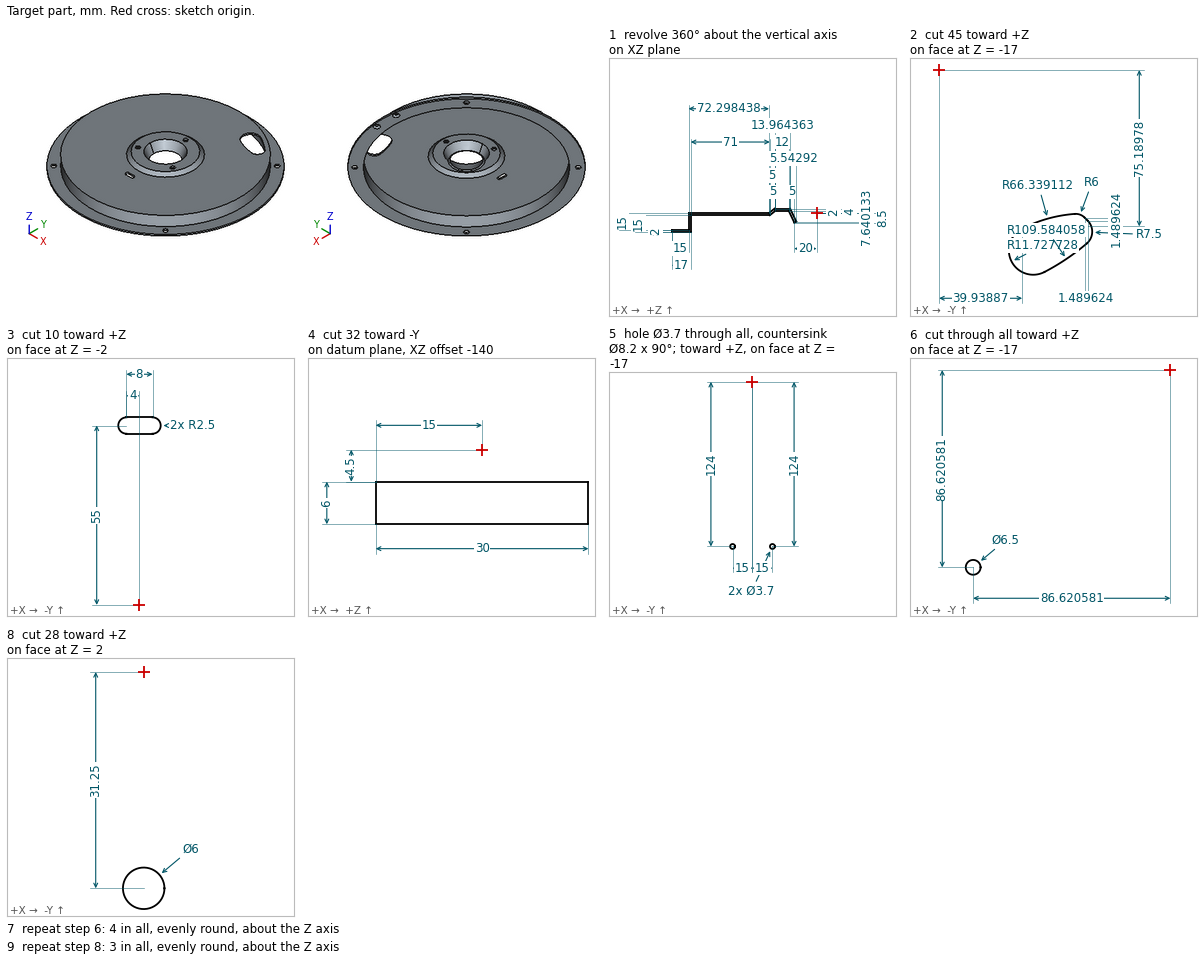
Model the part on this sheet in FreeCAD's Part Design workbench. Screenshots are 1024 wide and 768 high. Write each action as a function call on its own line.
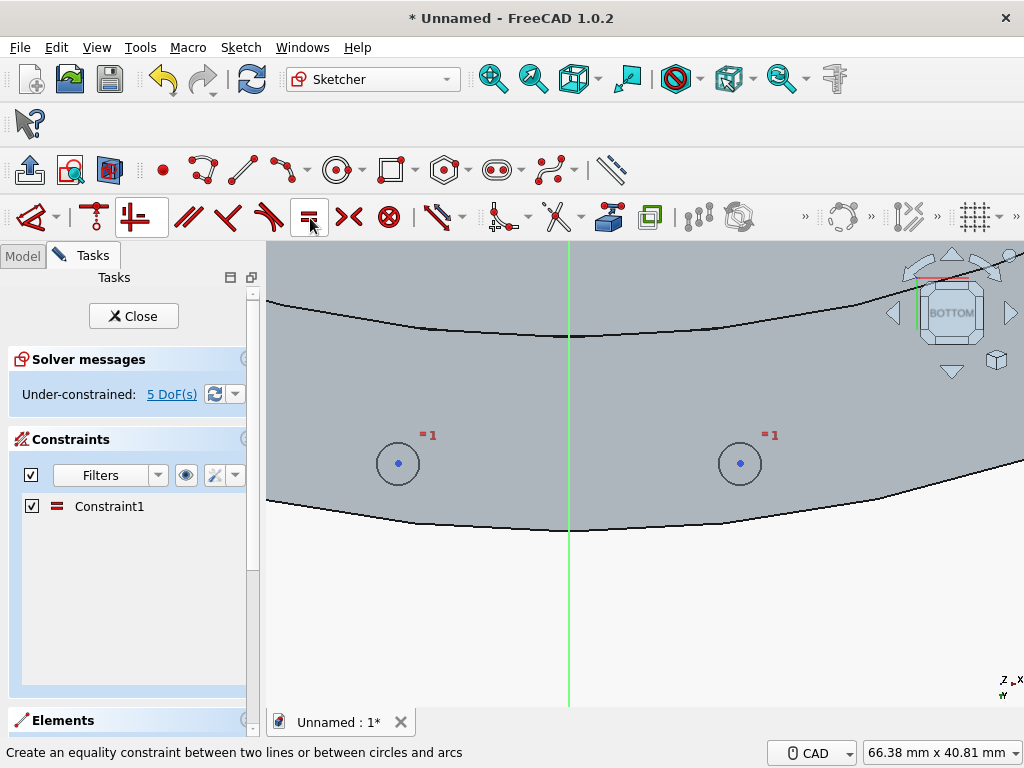
click(32, 218)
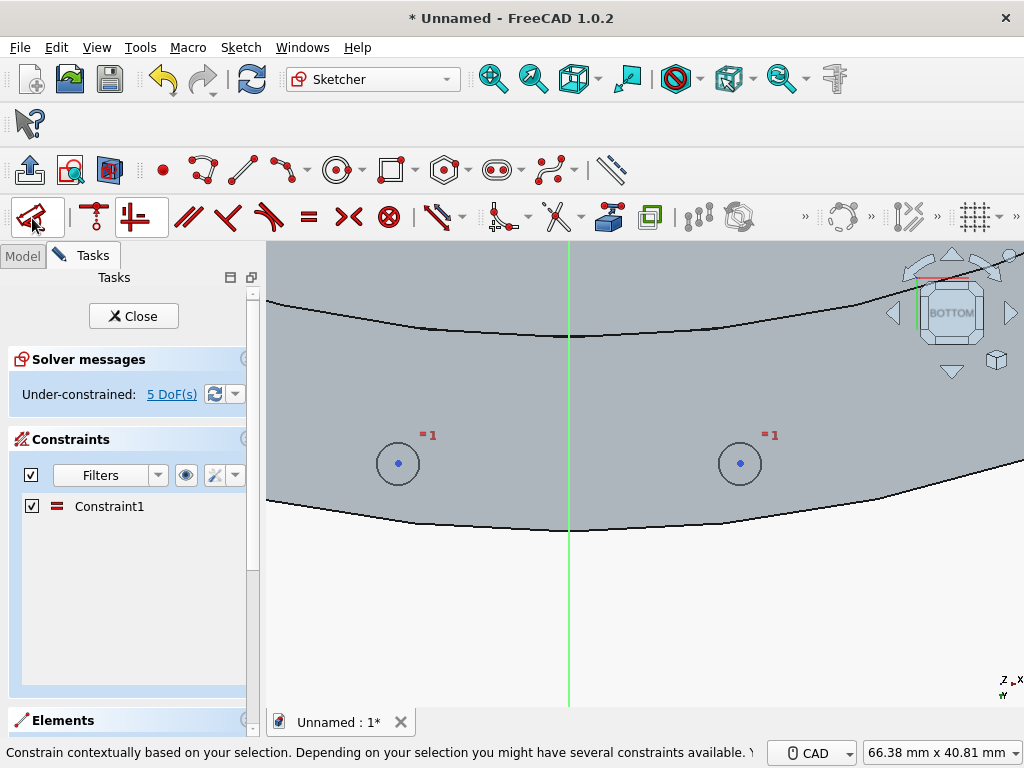
click(755, 449)
click(778, 426)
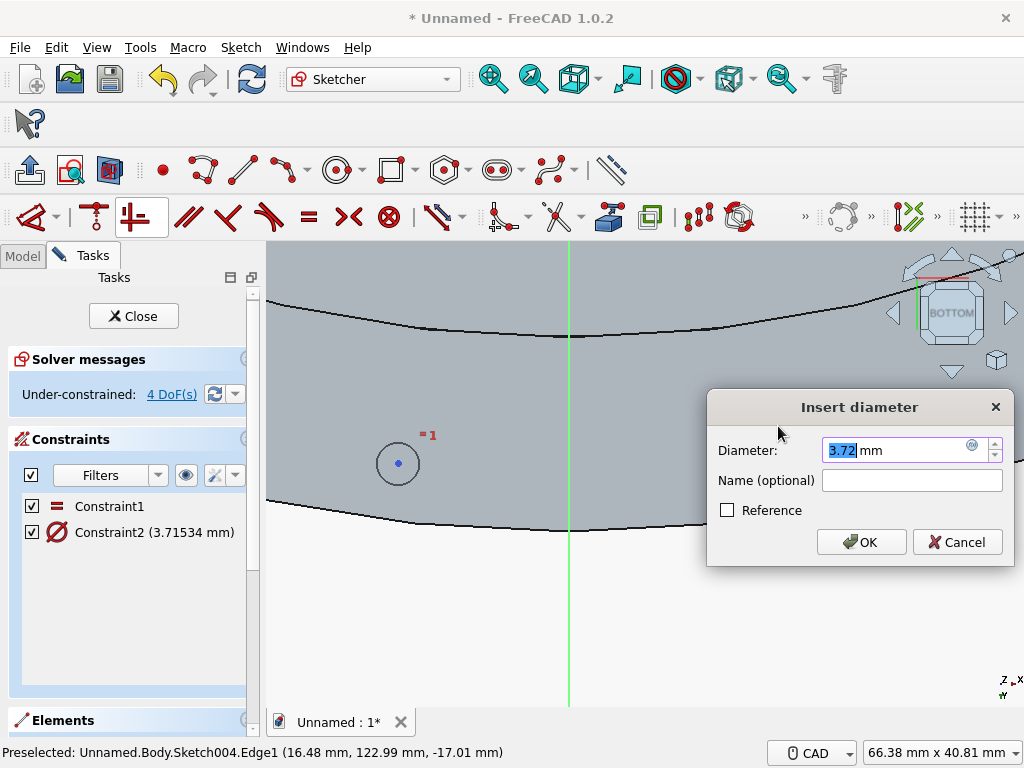
text(3.7)
key(Return)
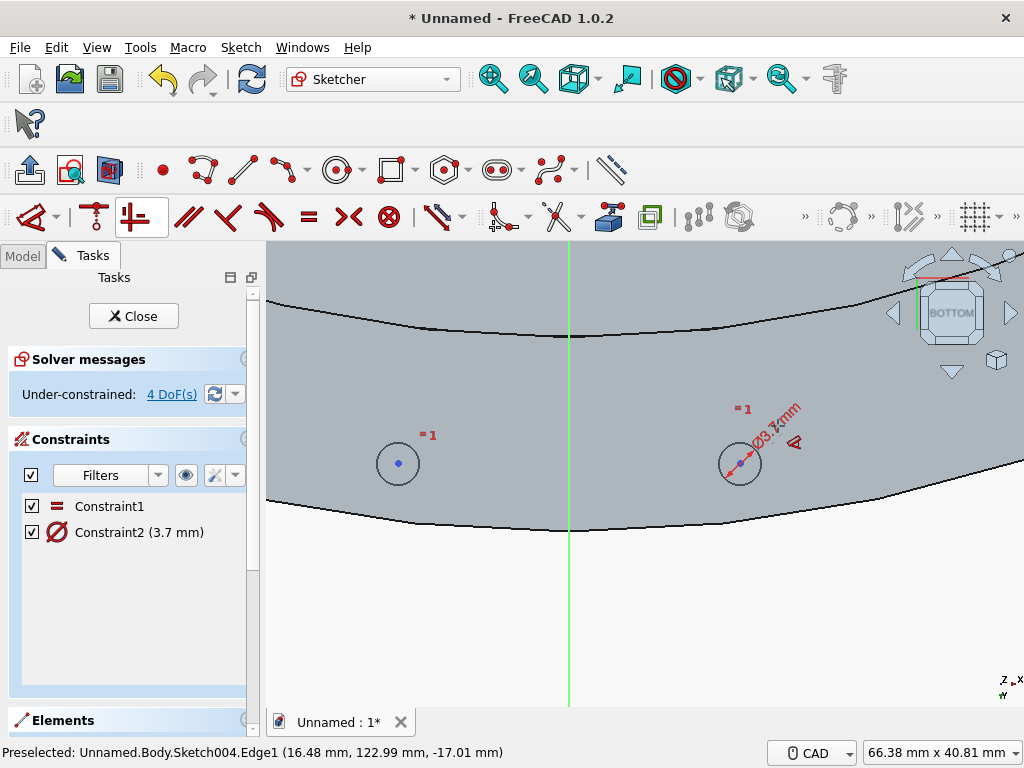
click(740, 464)
click(654, 498)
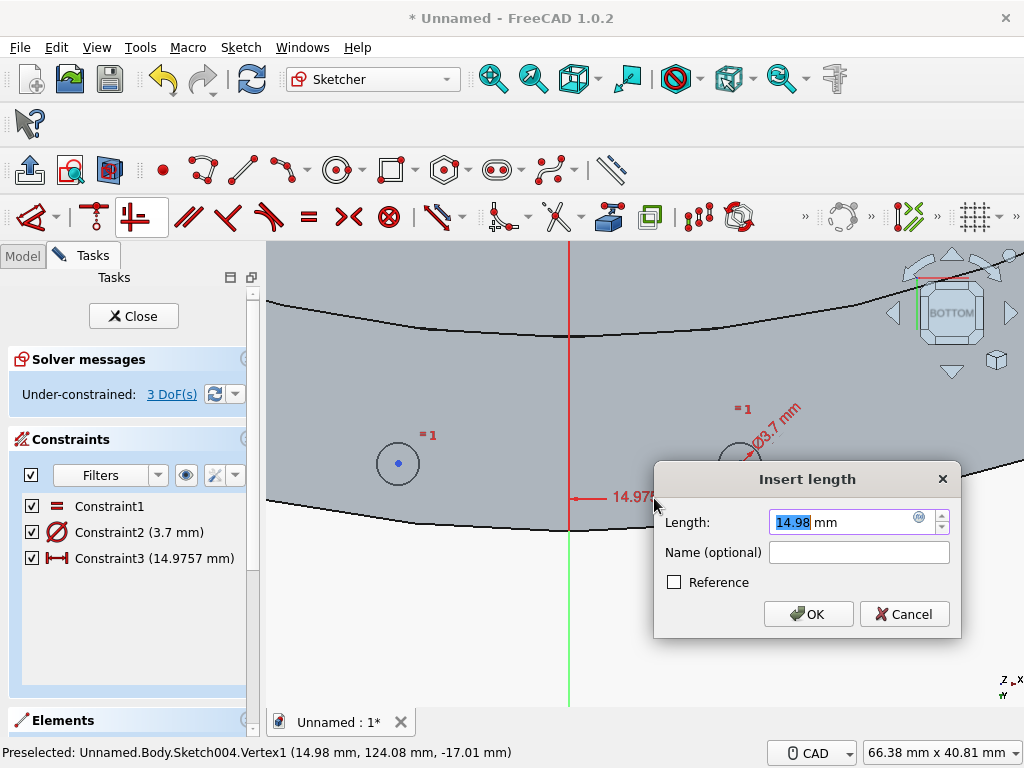
text(15)
key(Return)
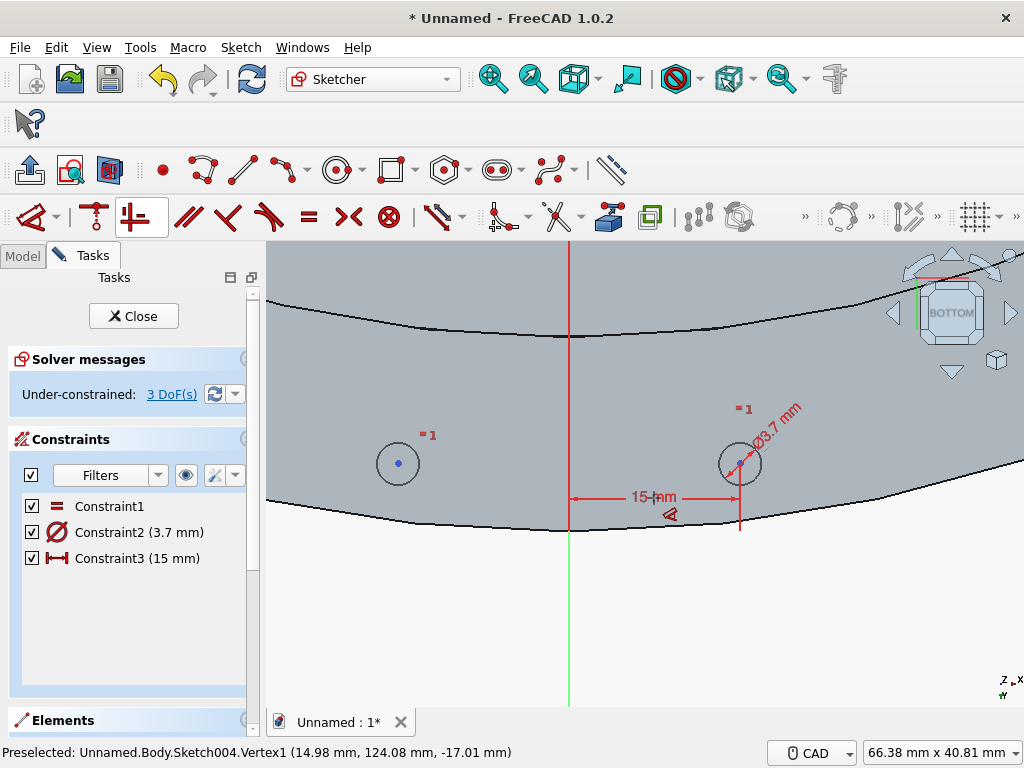
click(398, 464)
click(483, 498)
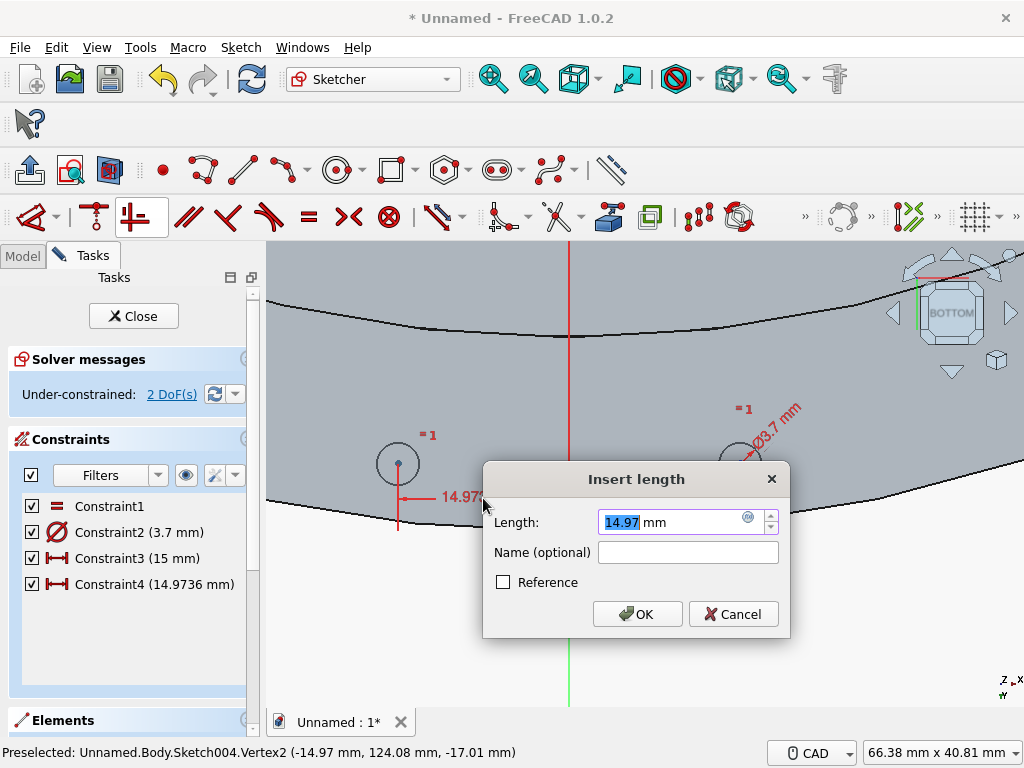
text(15)
key(Return)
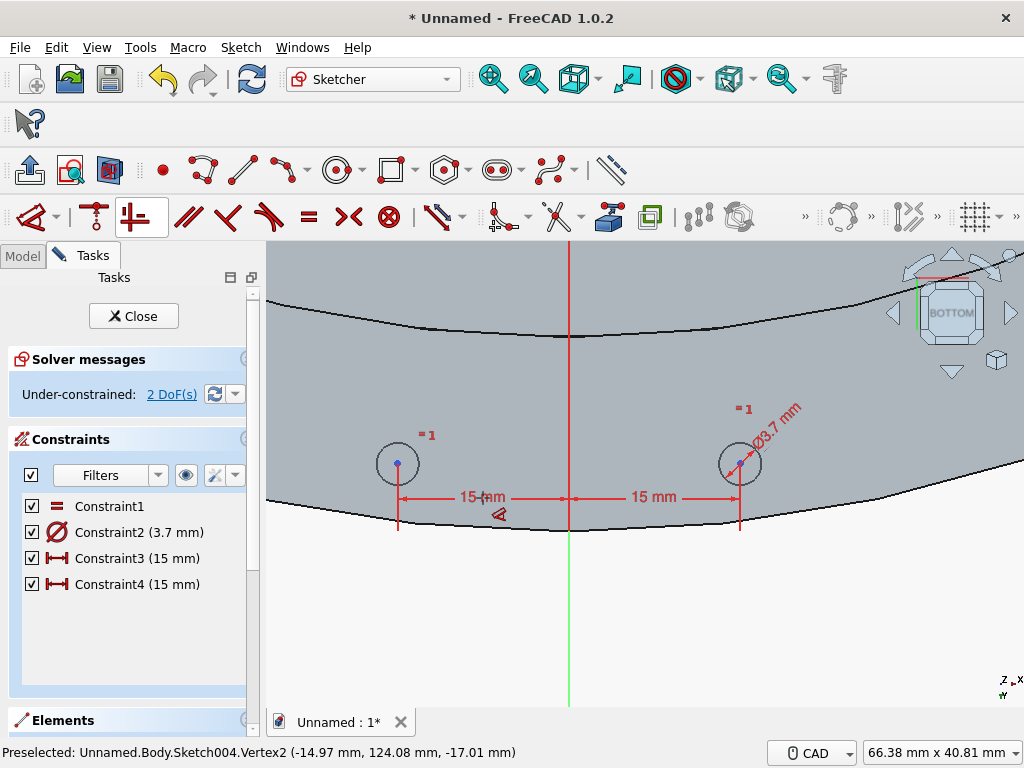
click(740, 464)
click(774, 367)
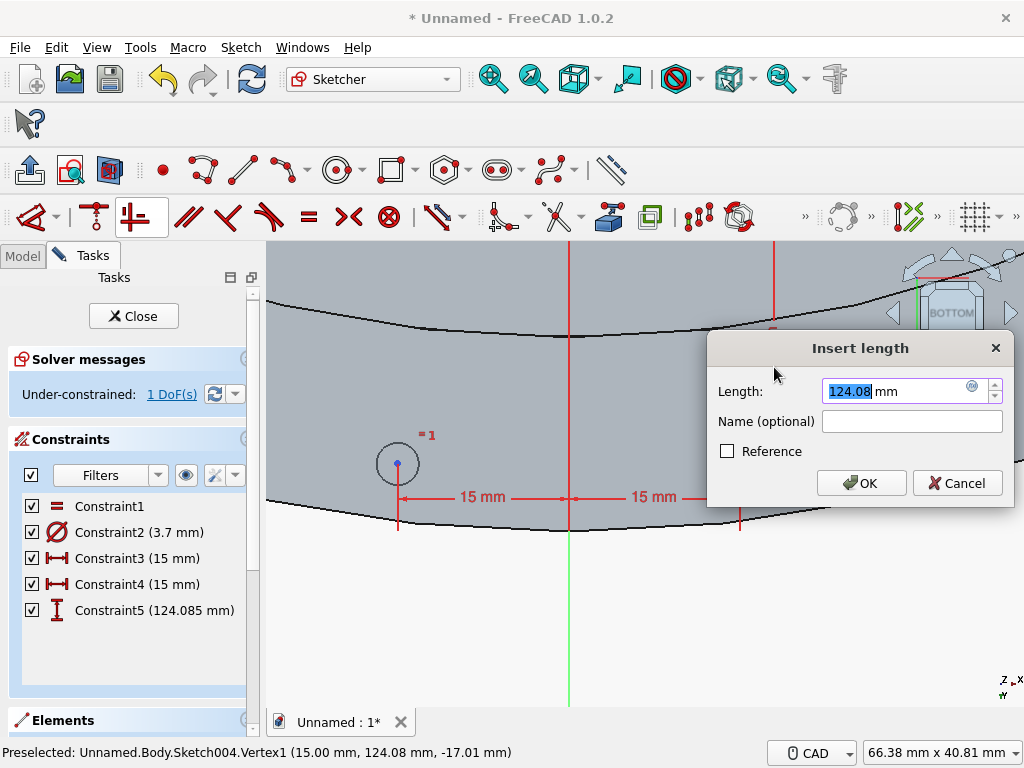
text(124)
key(Return)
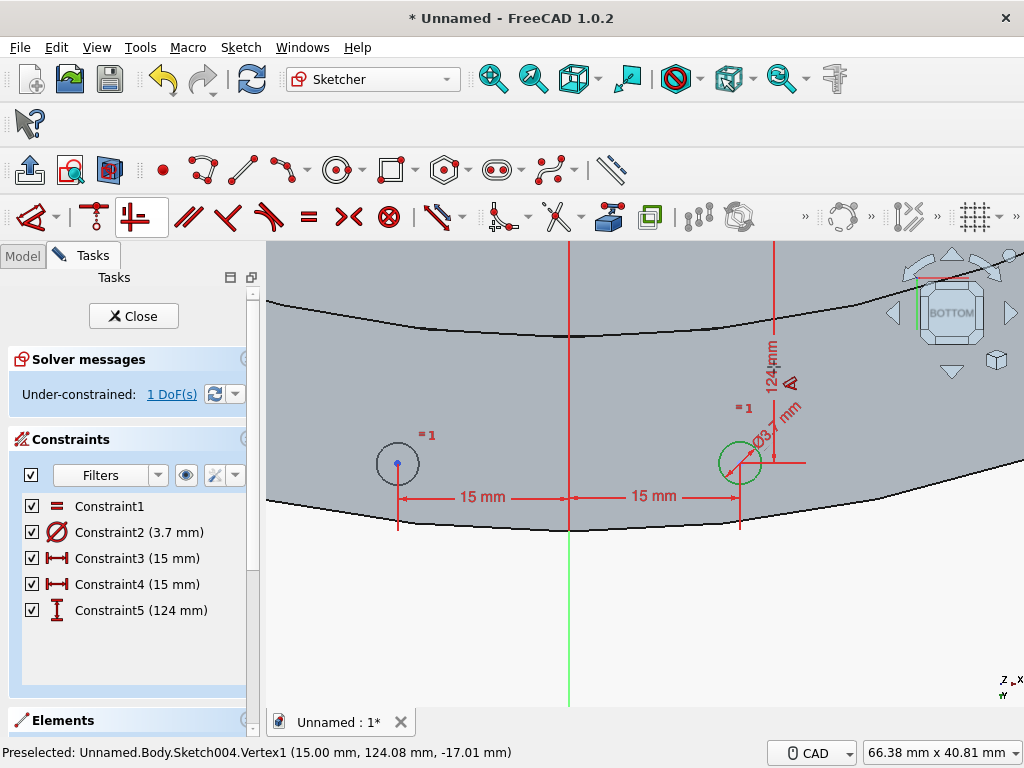
click(398, 464)
click(364, 367)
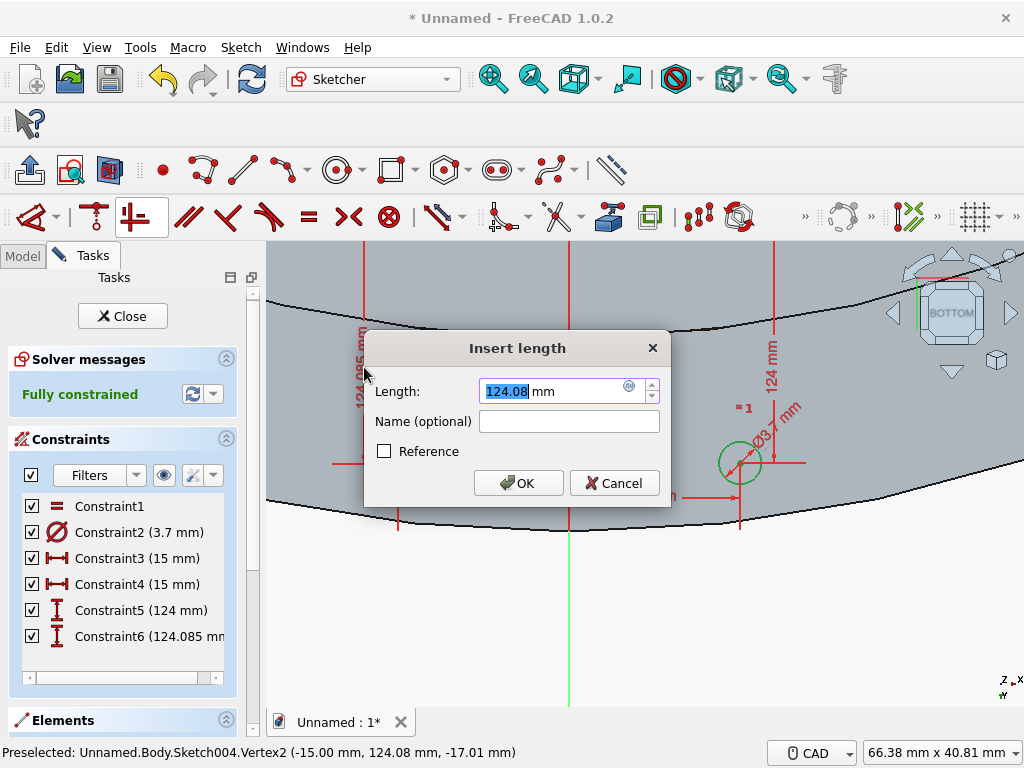
text(124)
key(Return)
key(Escape)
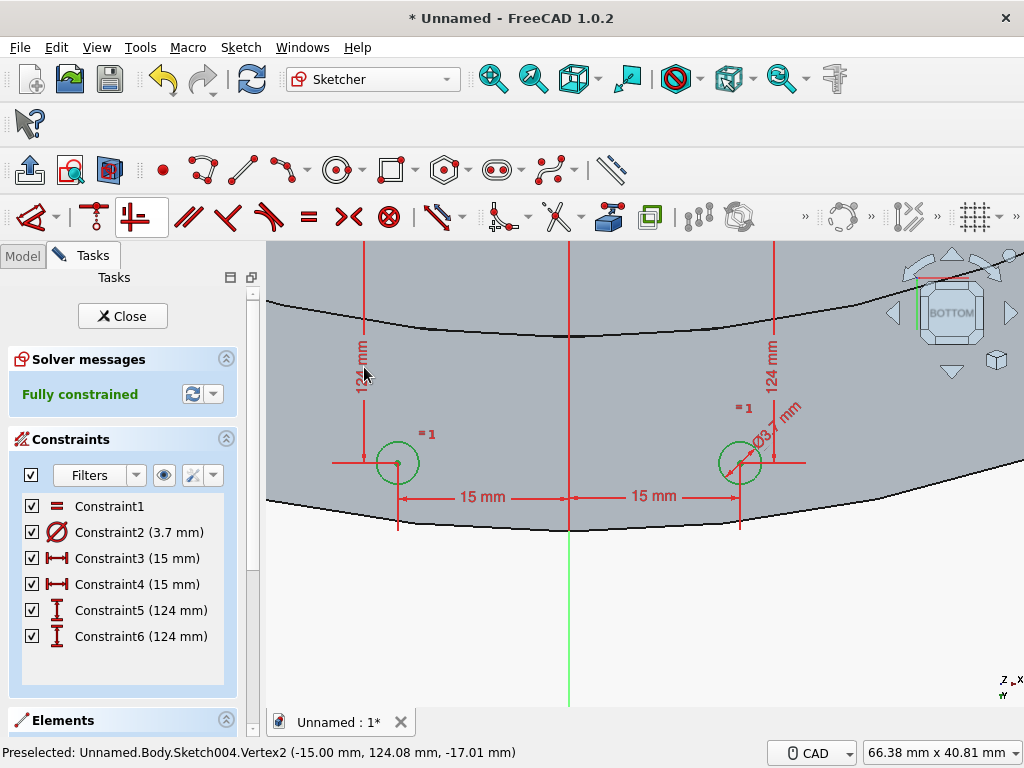
click(123, 316)